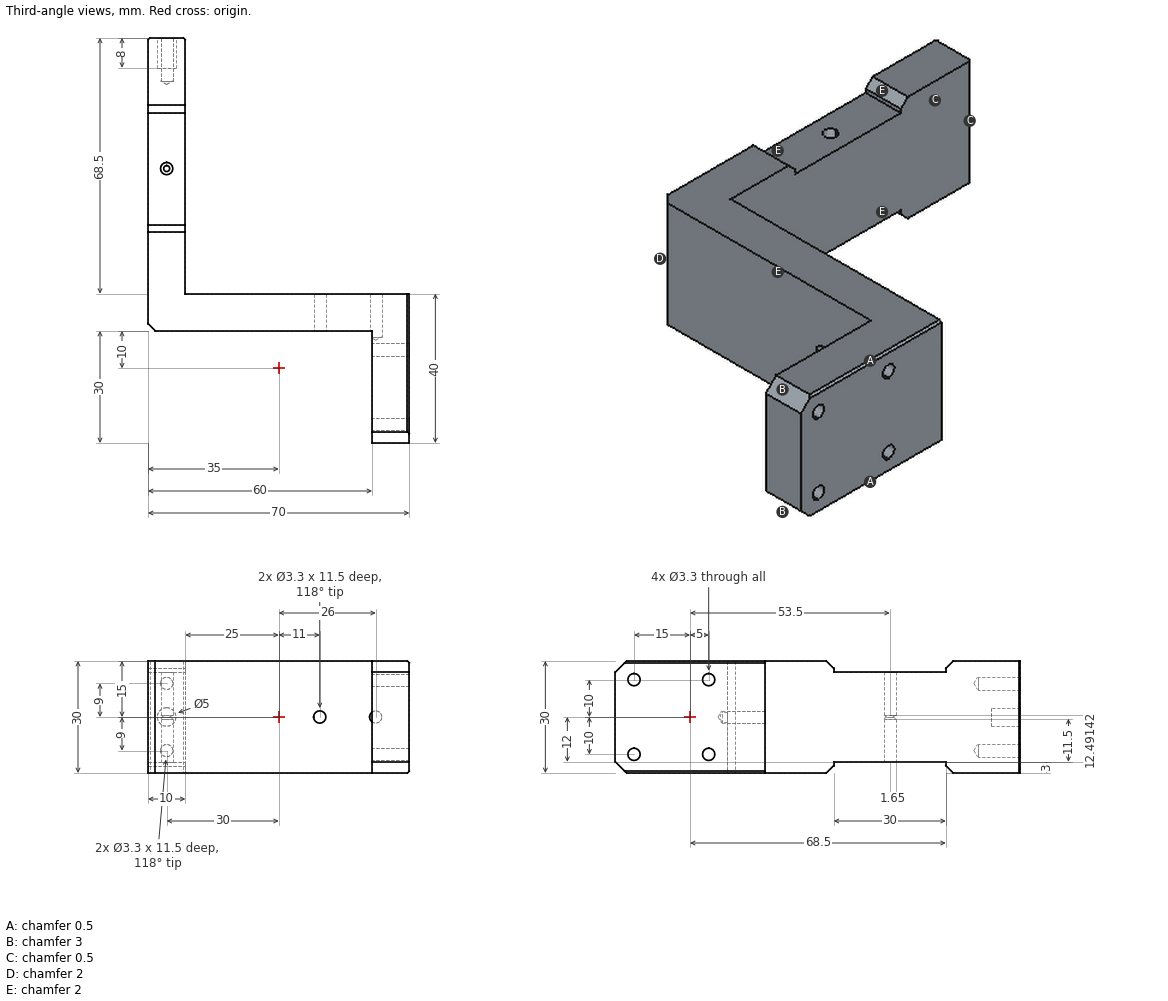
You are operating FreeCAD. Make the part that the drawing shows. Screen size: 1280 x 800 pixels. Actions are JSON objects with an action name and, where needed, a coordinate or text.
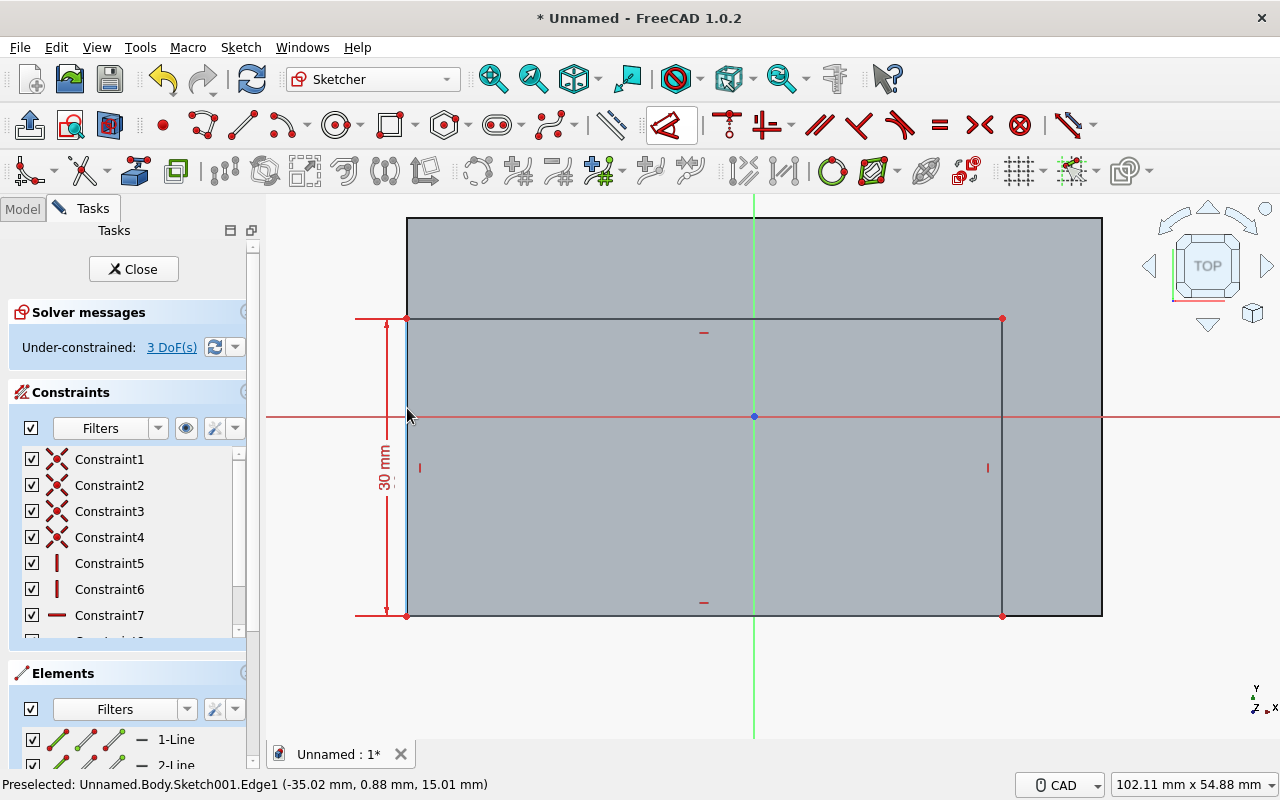
{"action": "left_click", "coordinate": [585, 616]}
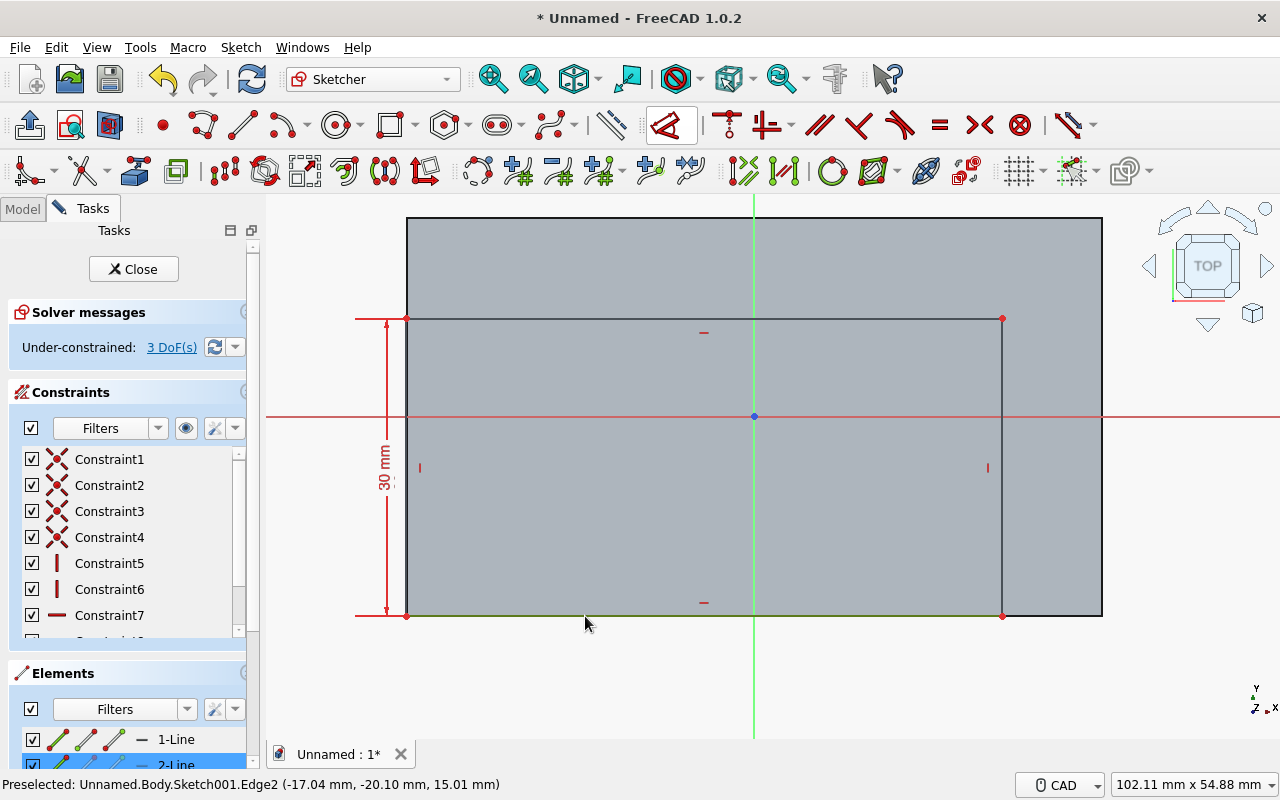
{"action": "key", "text": "l"}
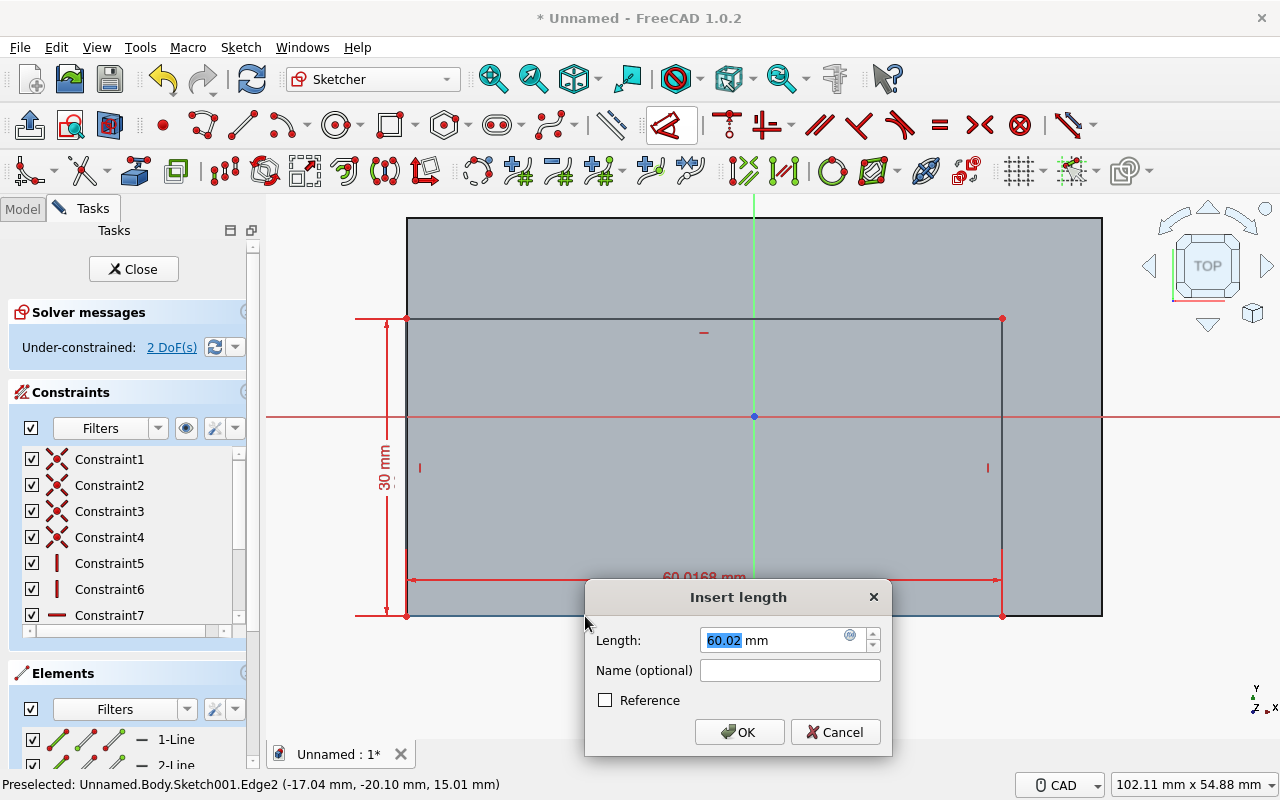
{"action": "type", "text": "60"}
{"action": "key", "text": "Return"}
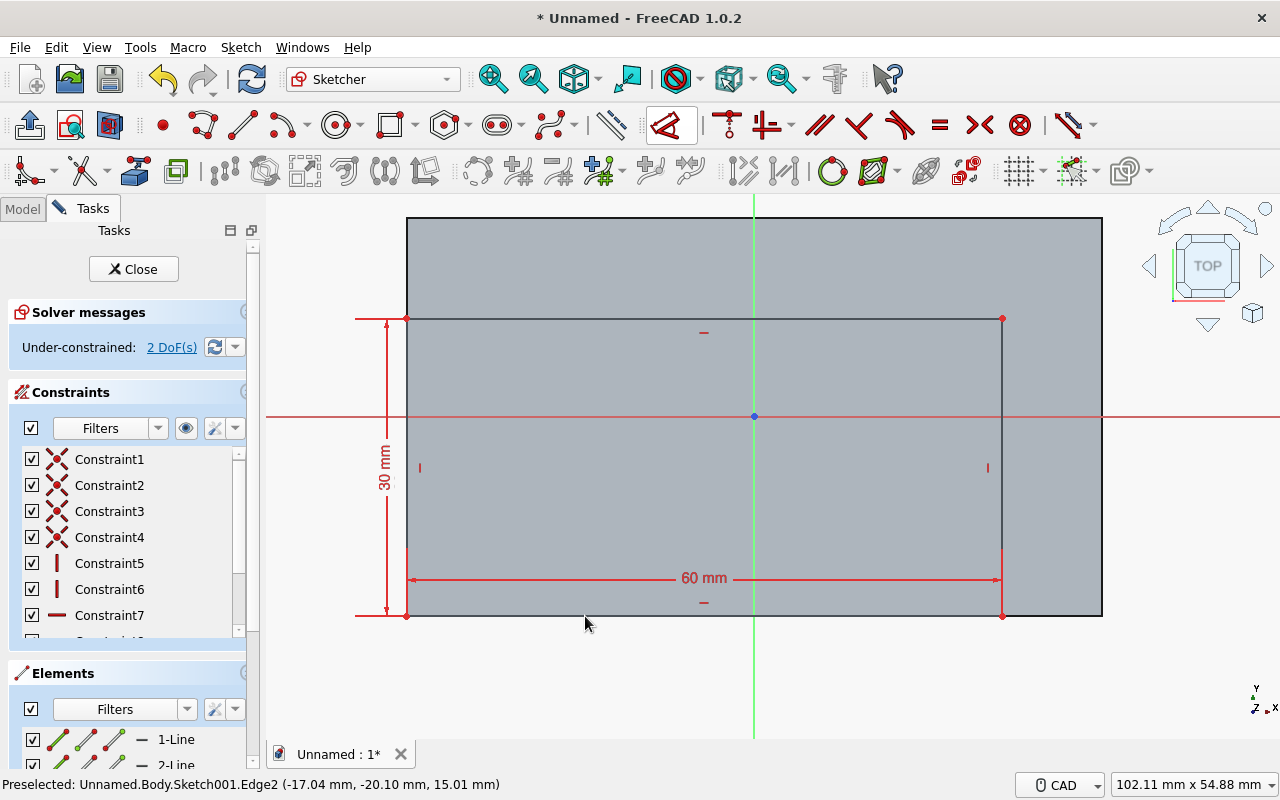
{"action": "left_click", "coordinate": [407, 319]}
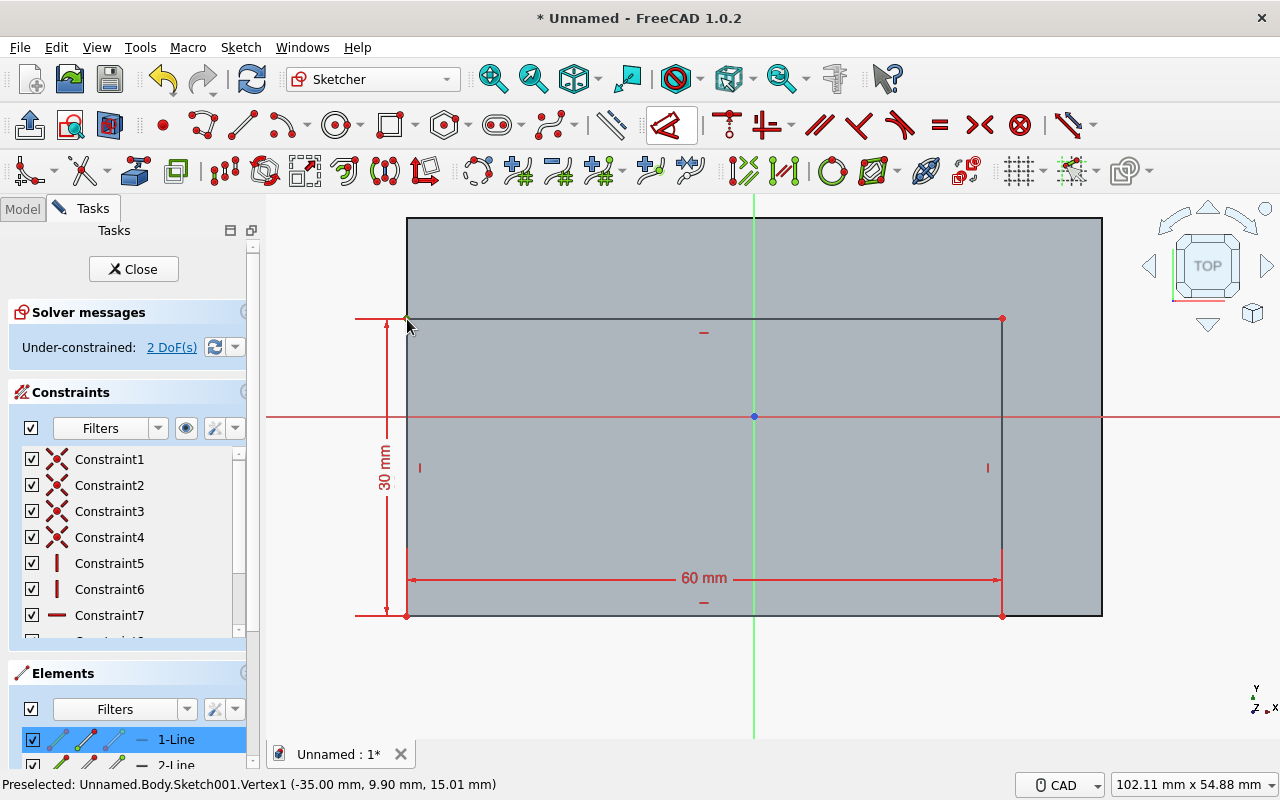
{"action": "left_click", "coordinate": [692, 126]}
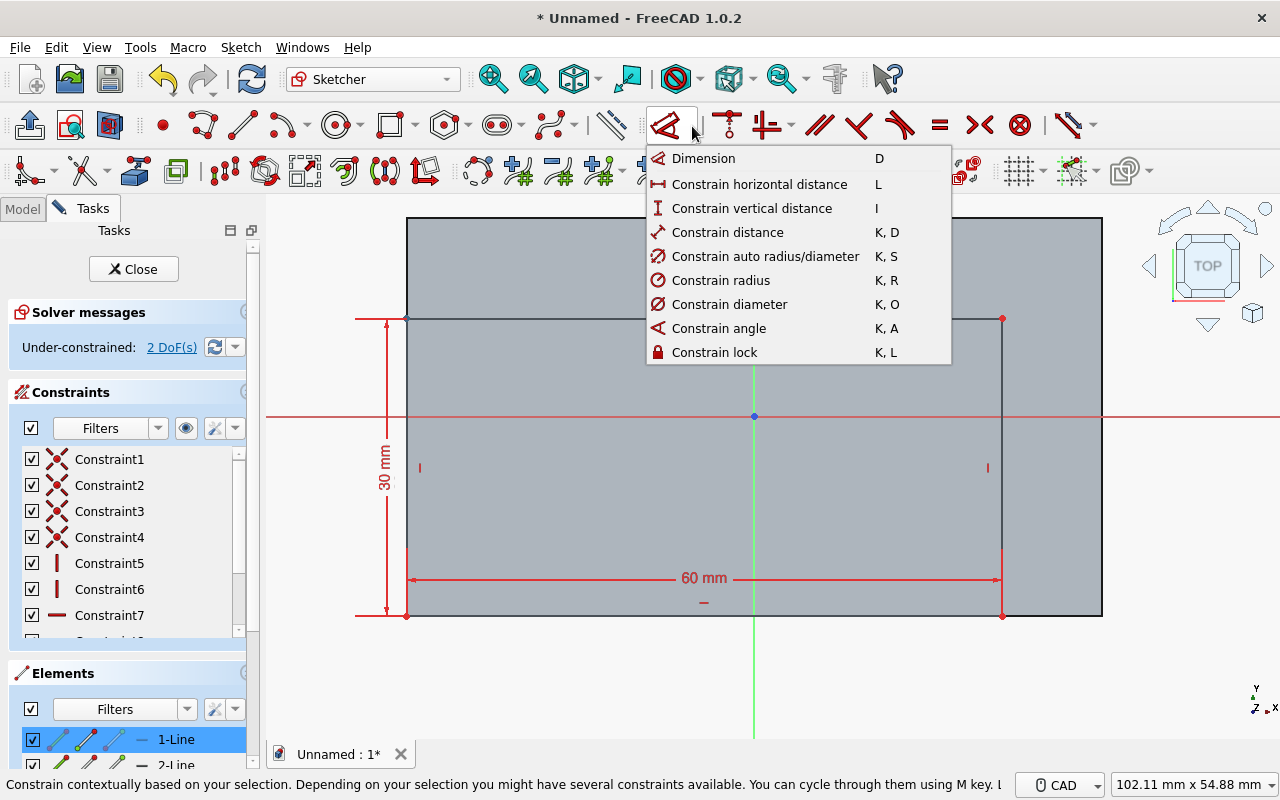
{"action": "left_click", "coordinate": [799, 184]}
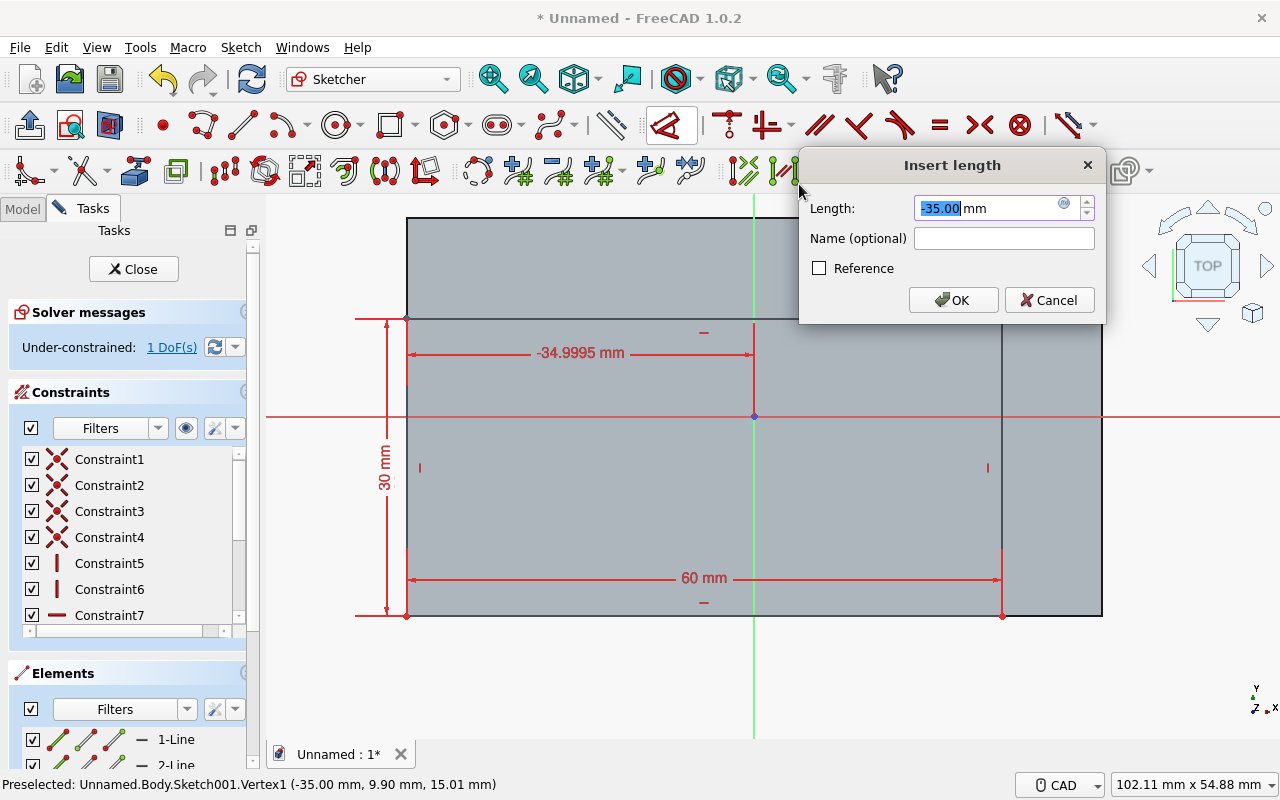
{"action": "type", "text": "-35"}
{"action": "key", "text": "Return"}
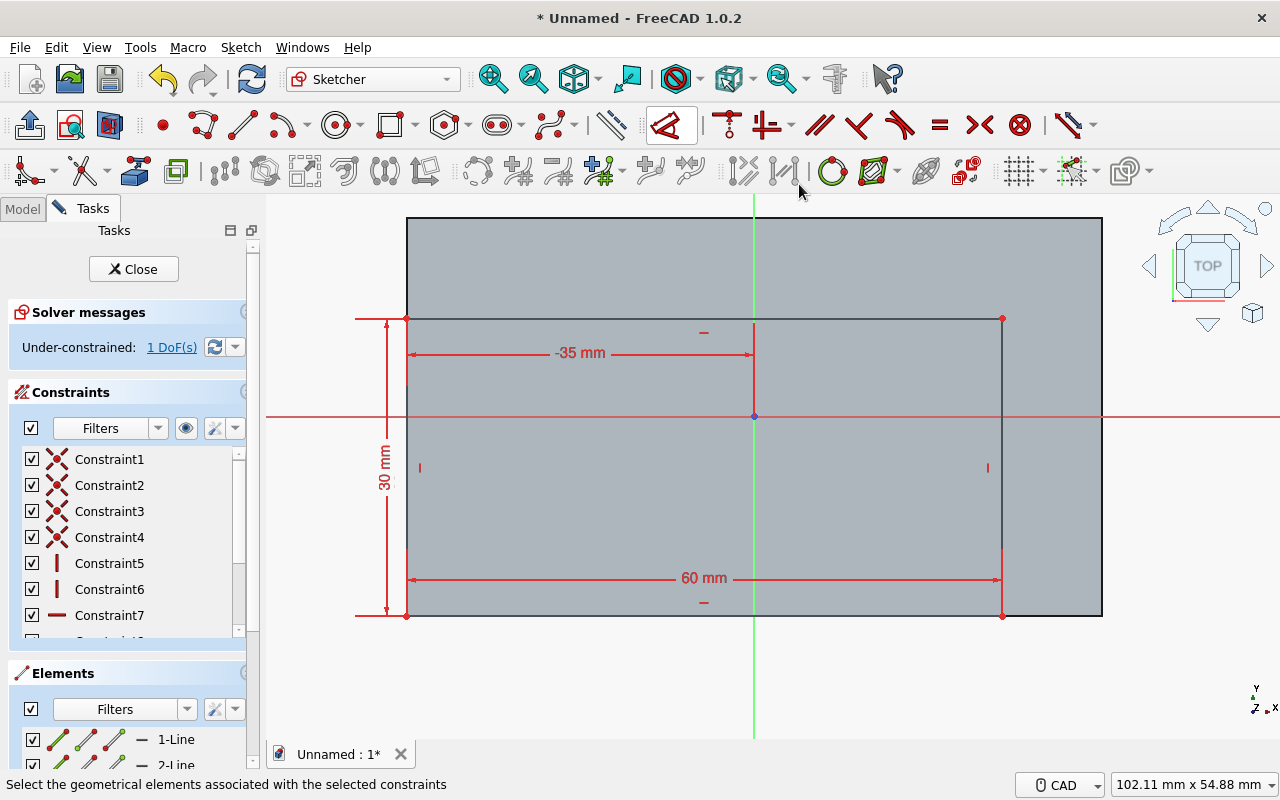
{"action": "left_click", "coordinate": [407, 319]}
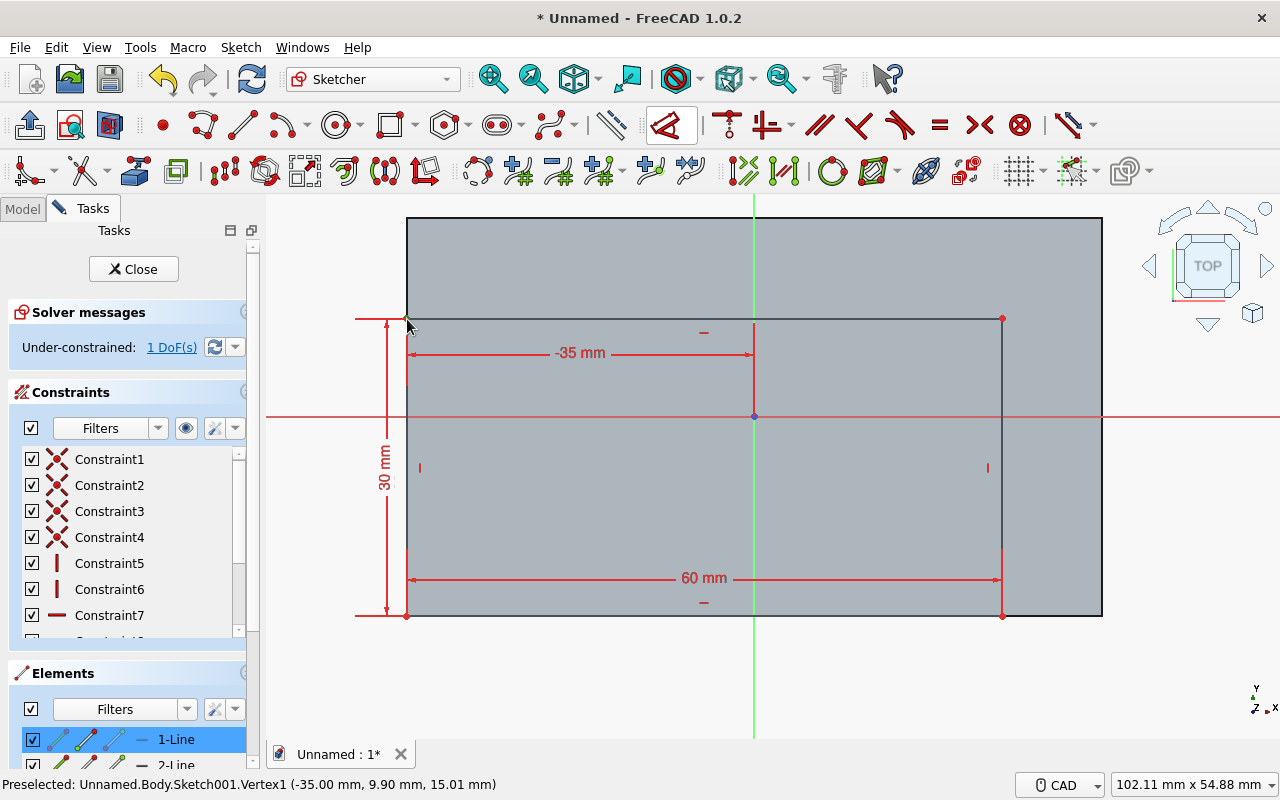
{"action": "left_click", "coordinate": [692, 126]}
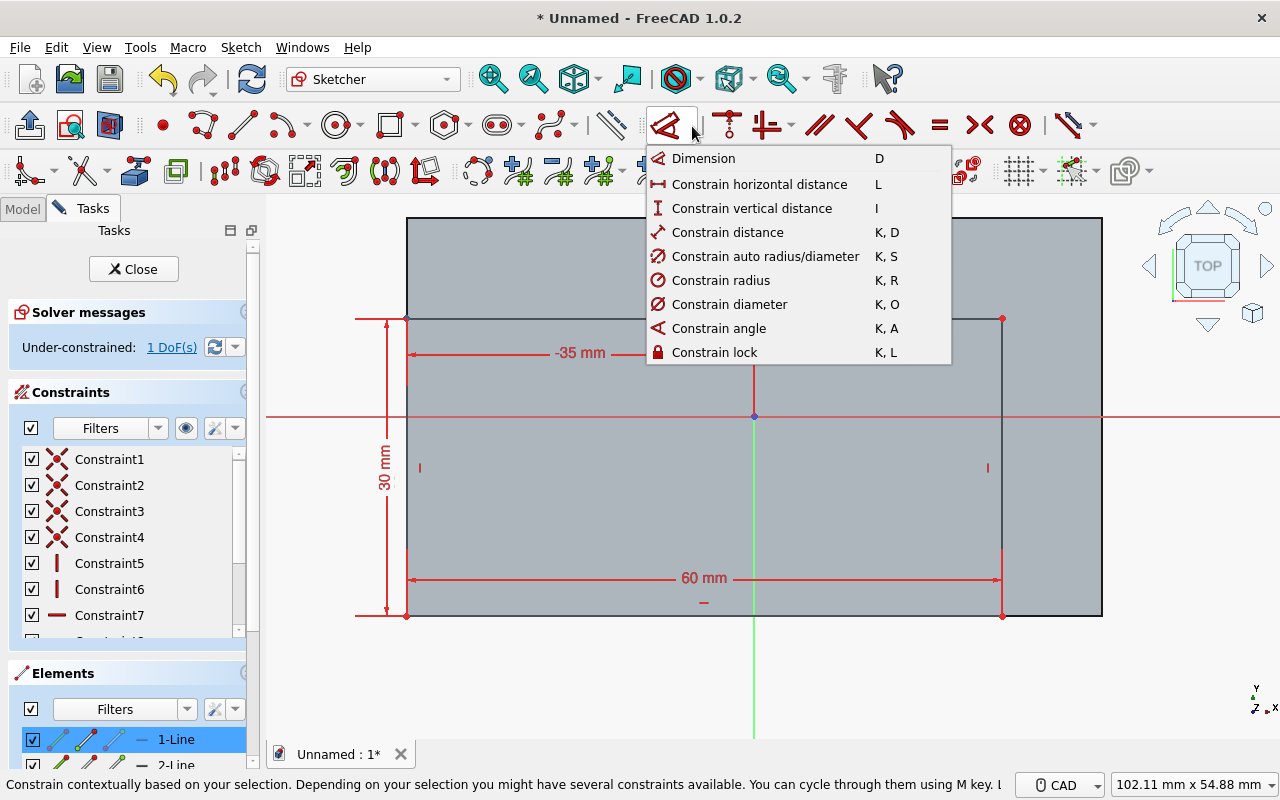
{"action": "left_click", "coordinate": [799, 208]}